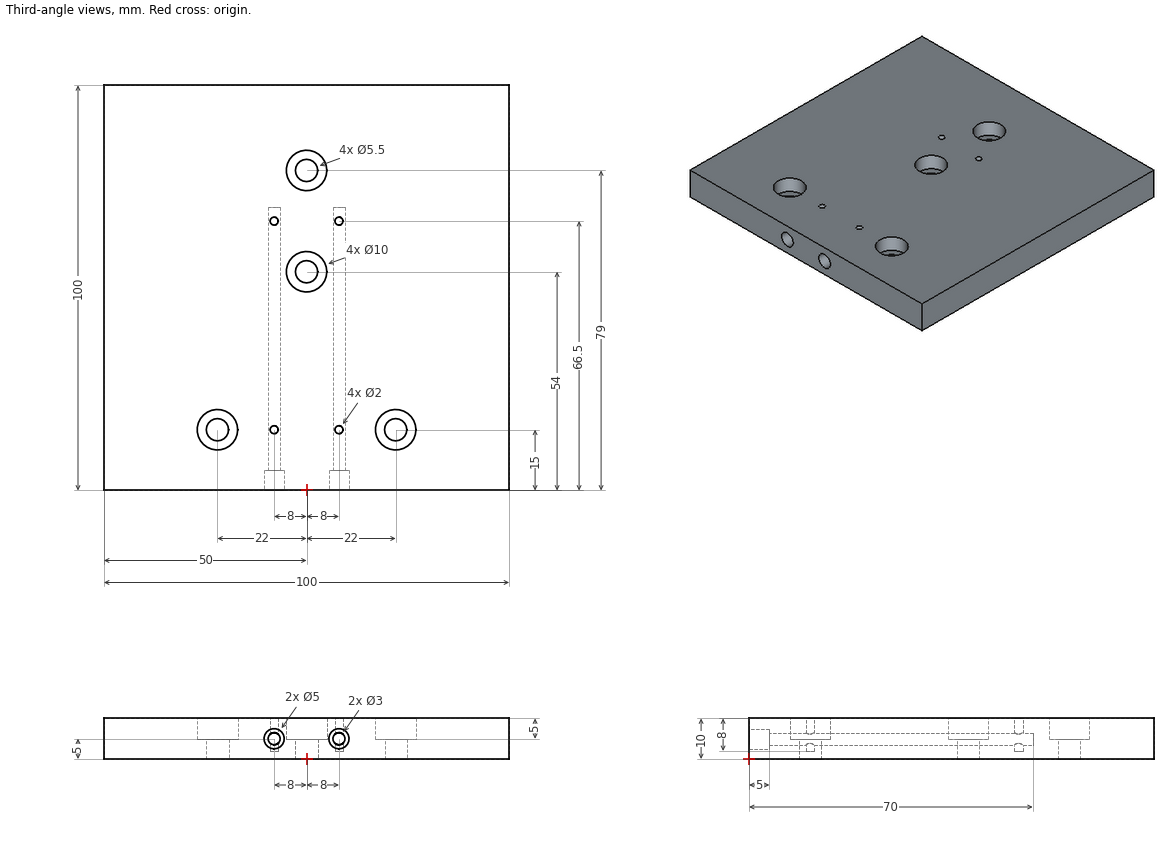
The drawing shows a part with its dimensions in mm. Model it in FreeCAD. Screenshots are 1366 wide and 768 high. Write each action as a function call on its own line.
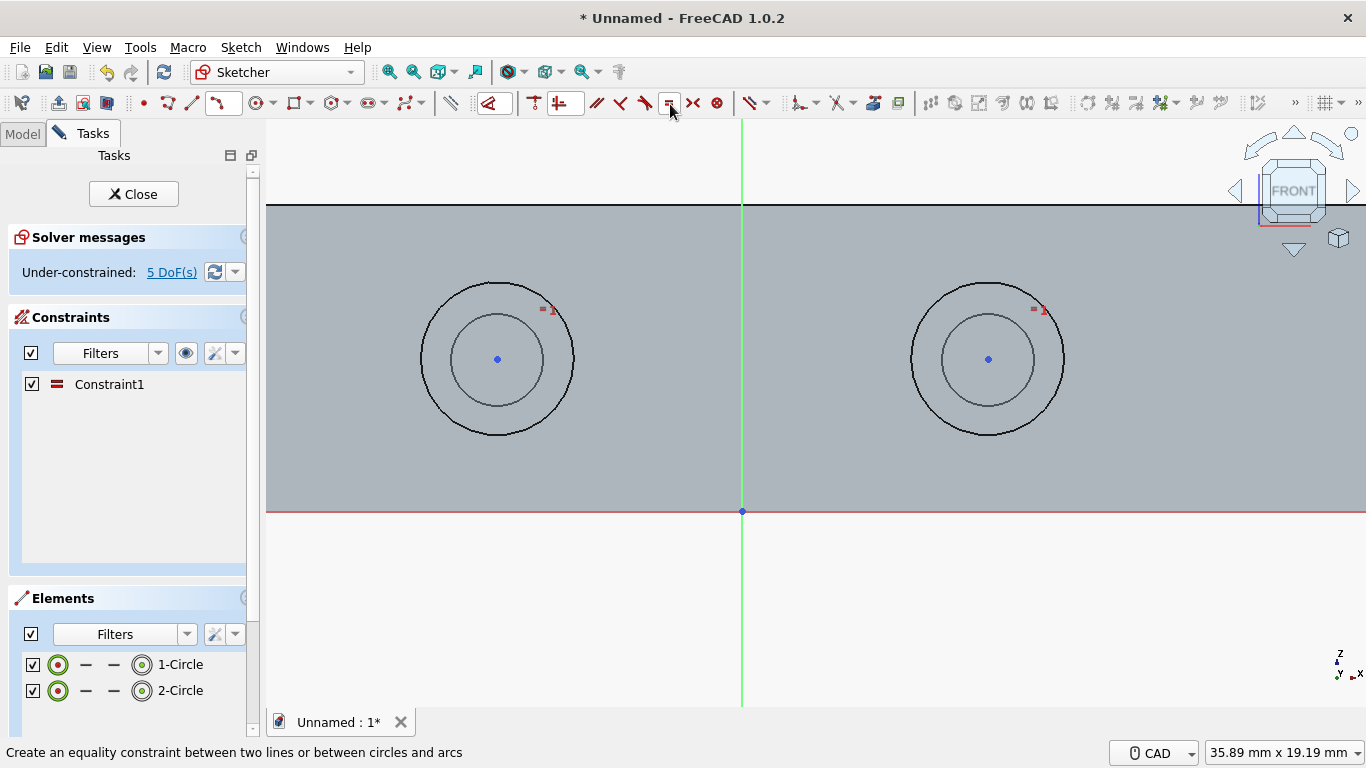
click(1020, 327)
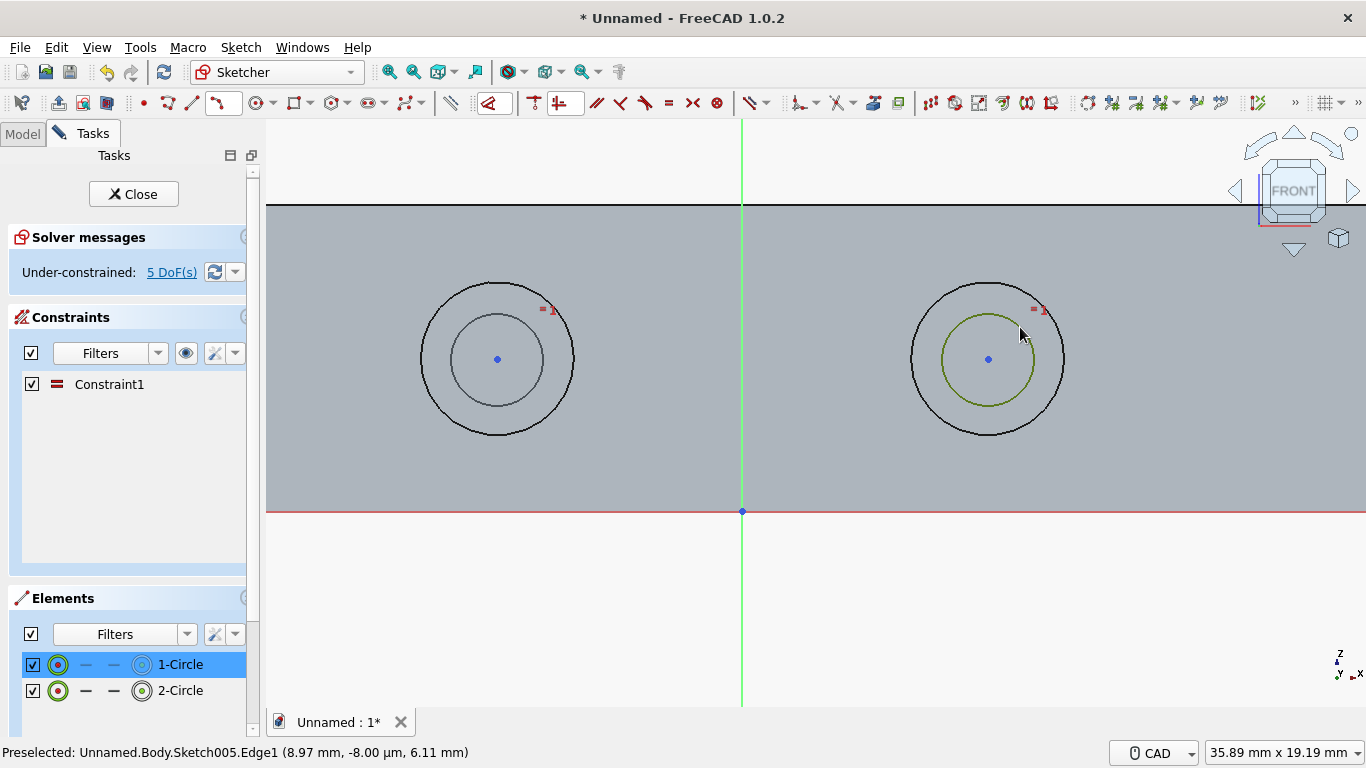
key(k)
key(o)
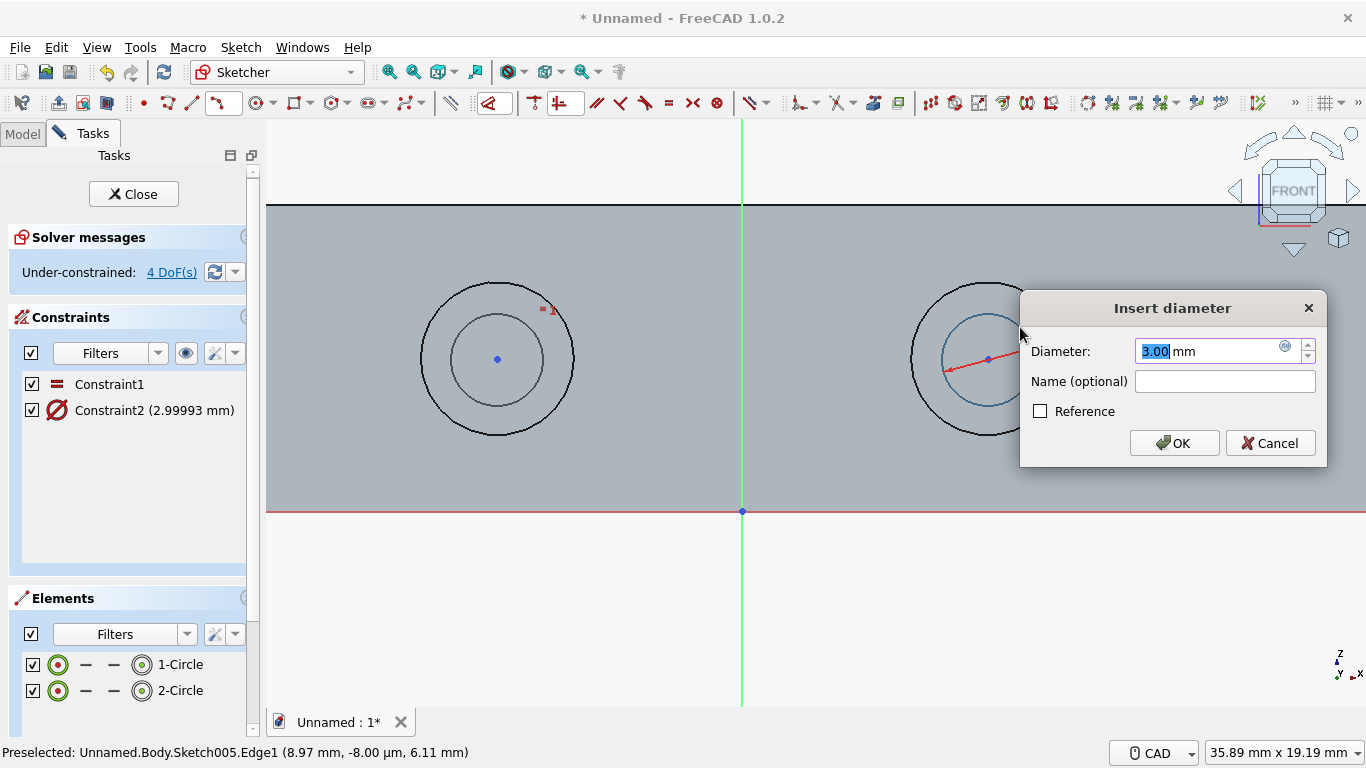
text(3)
key(Return)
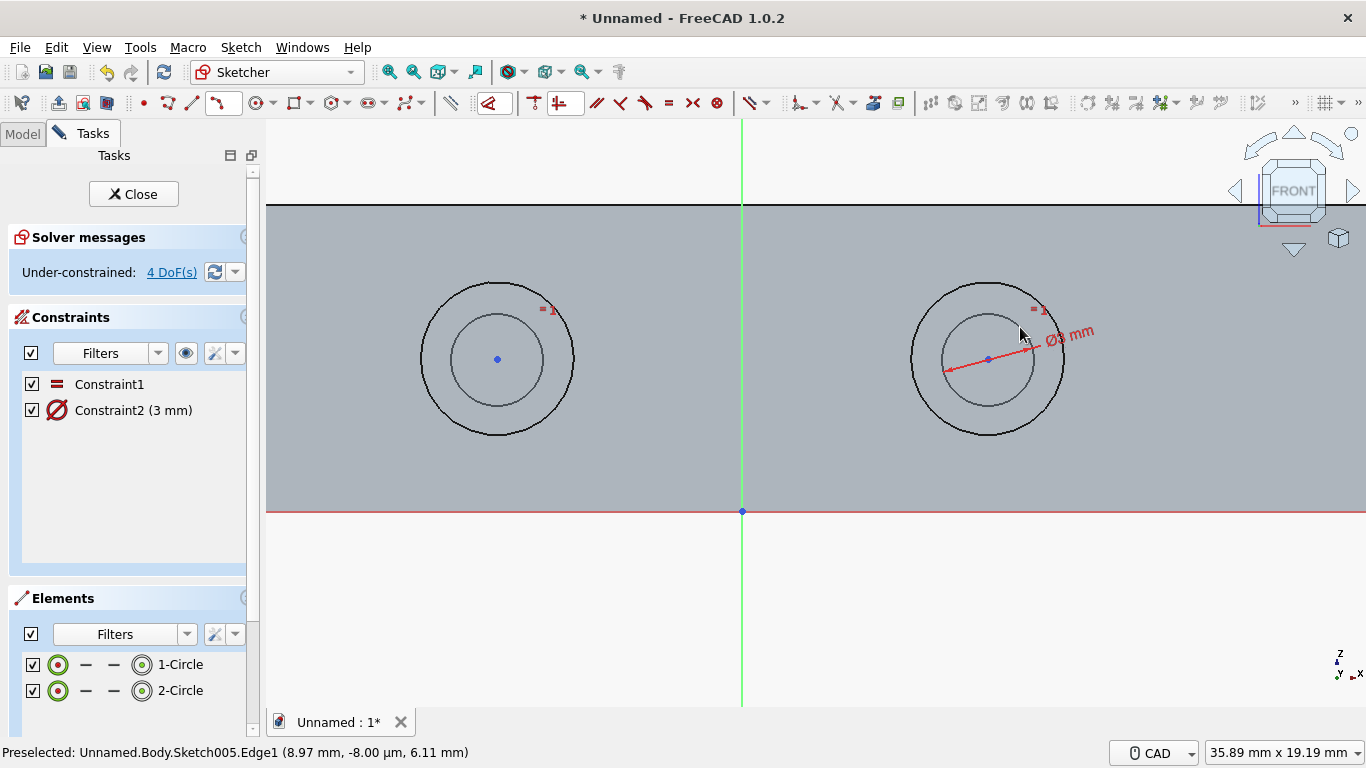
click(988, 360)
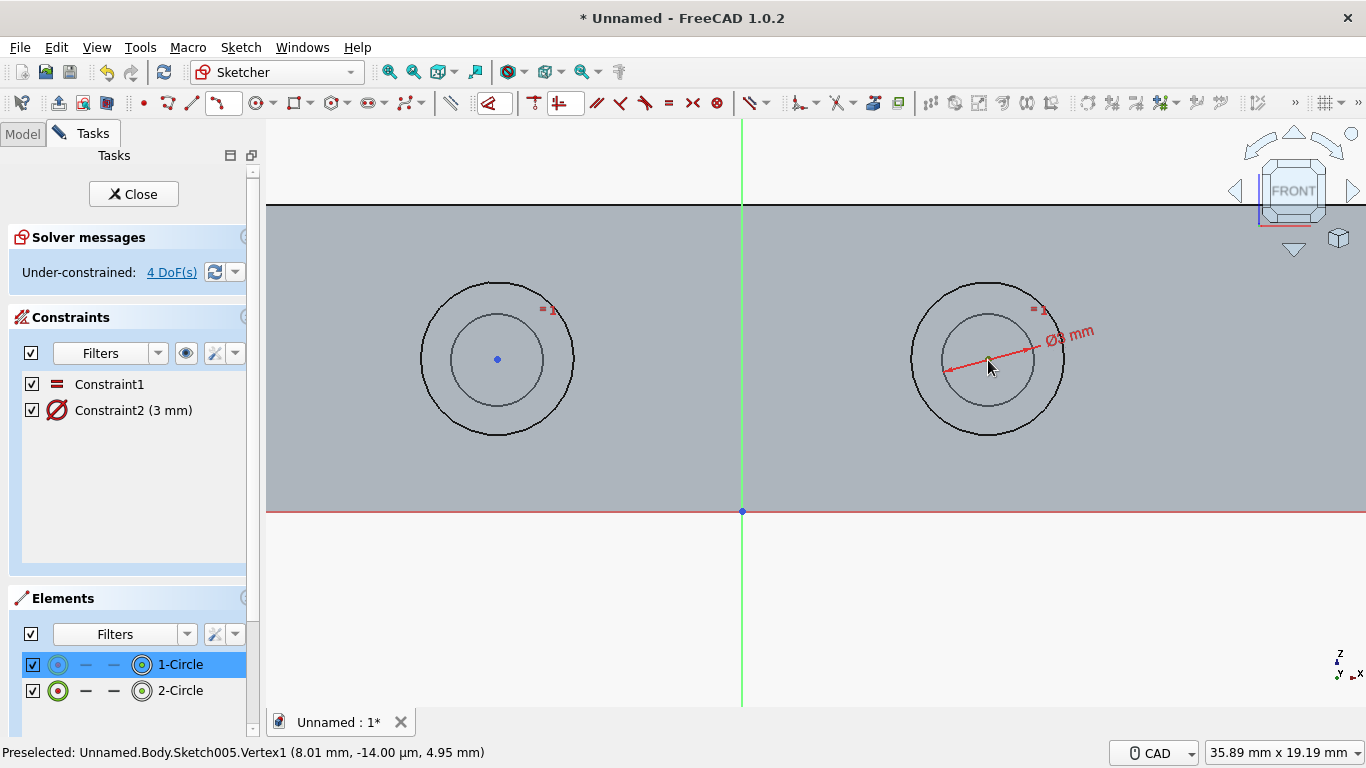
key(l)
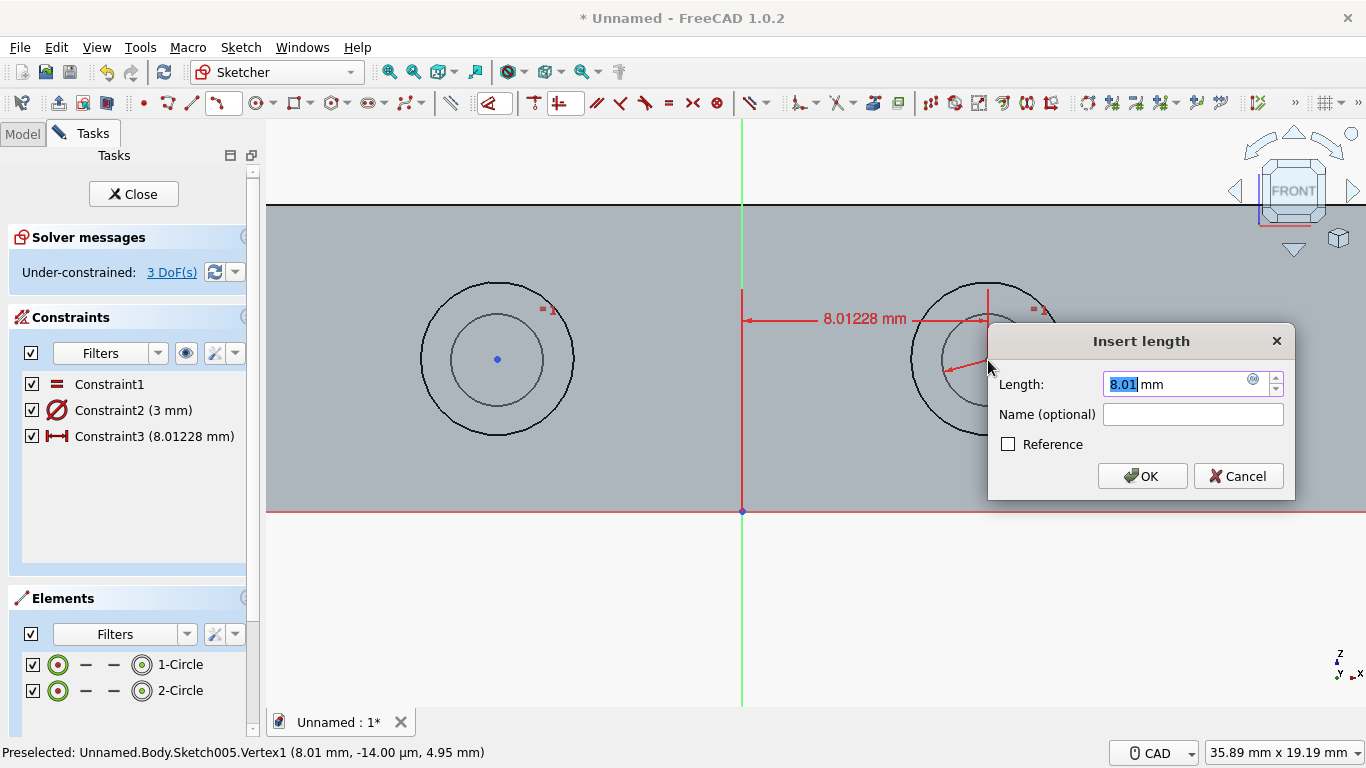
text(8)
key(Return)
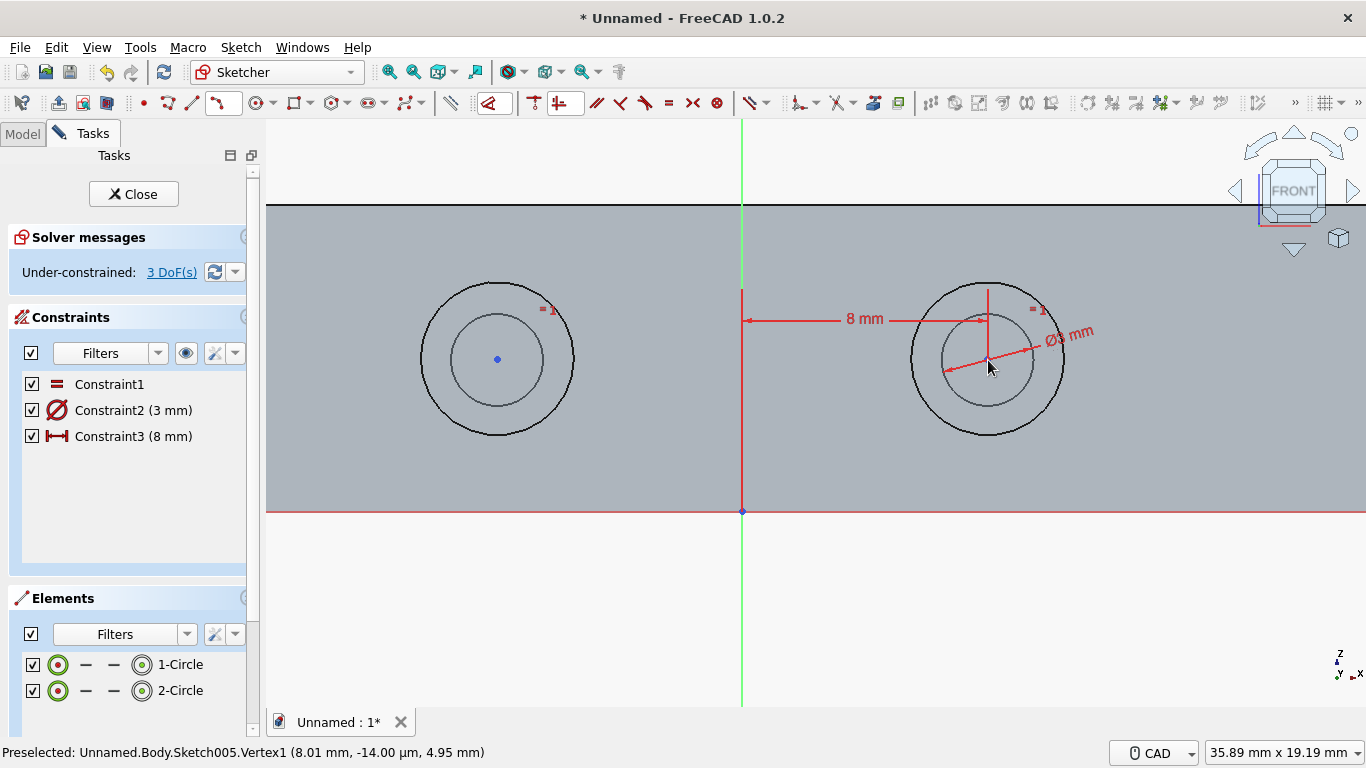
click(988, 360)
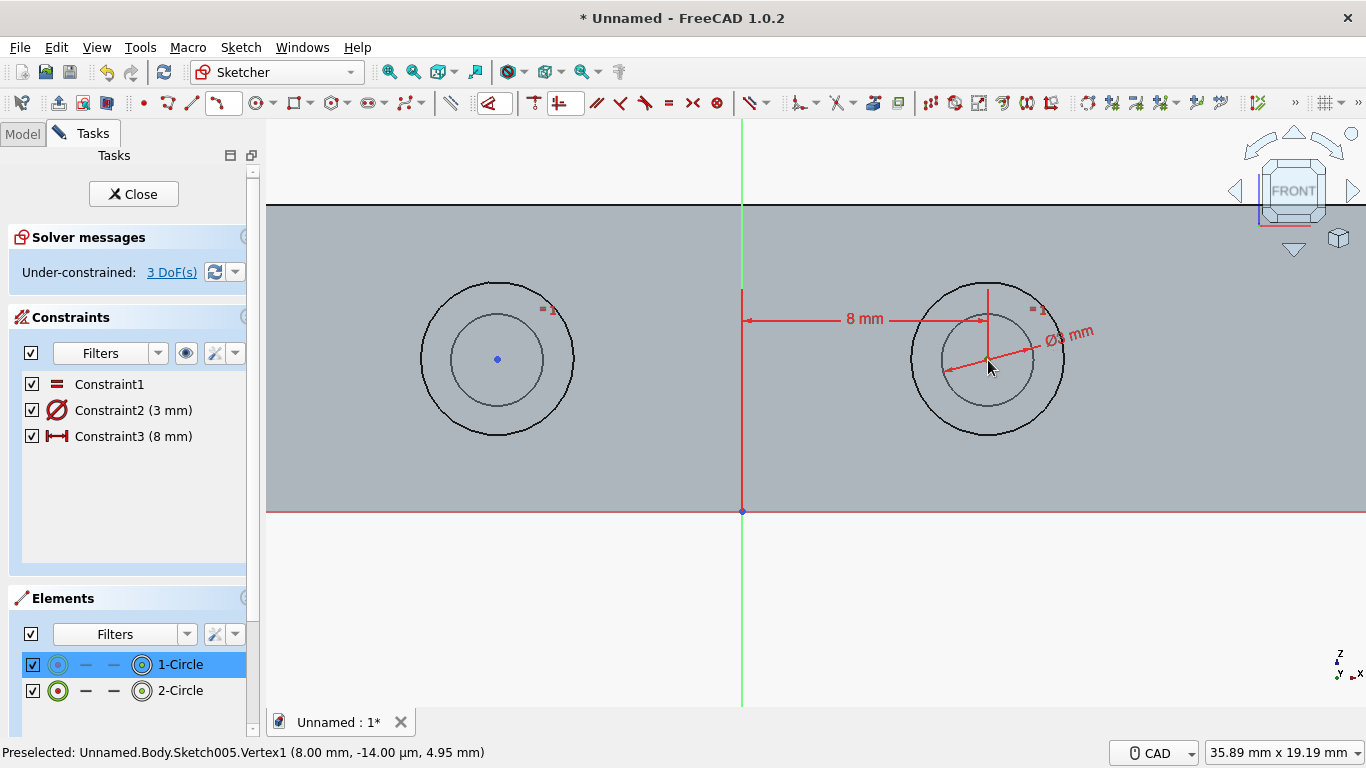
click(506, 104)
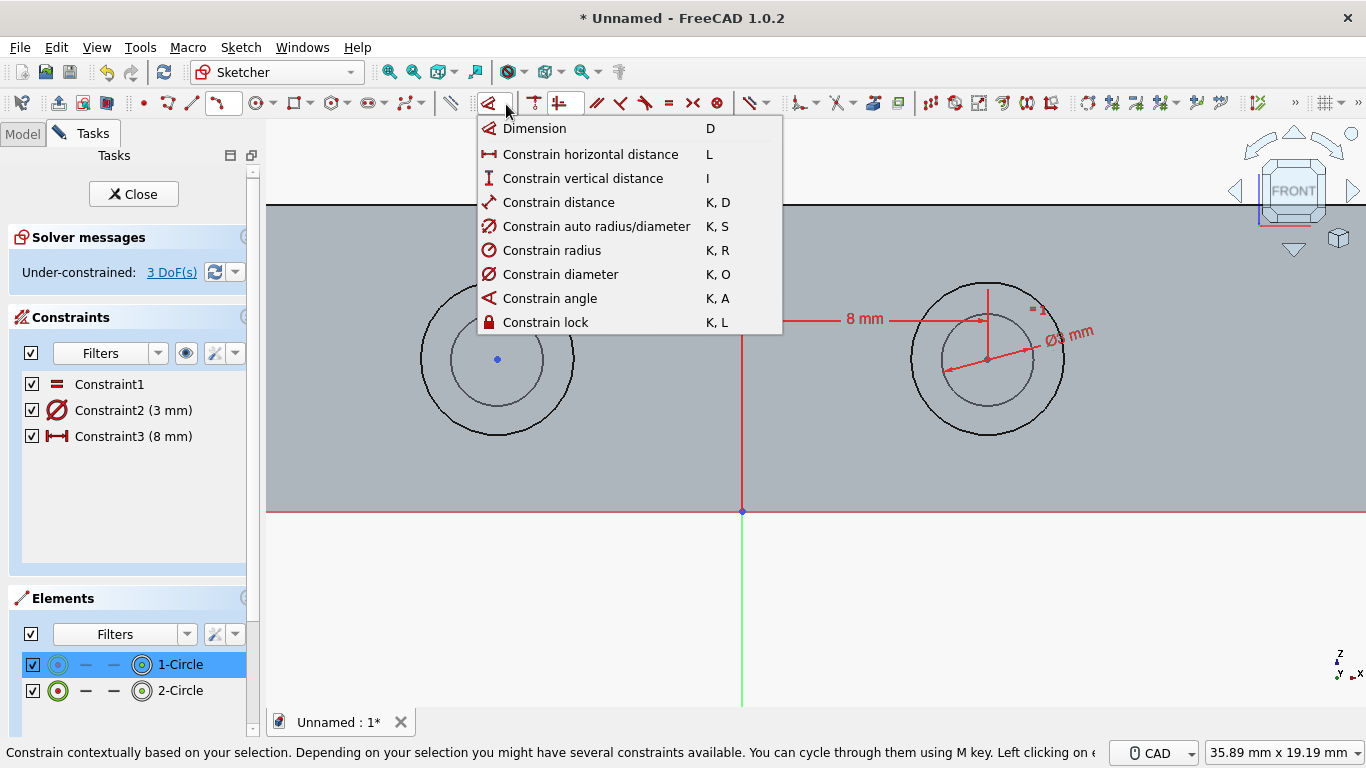
click(630, 178)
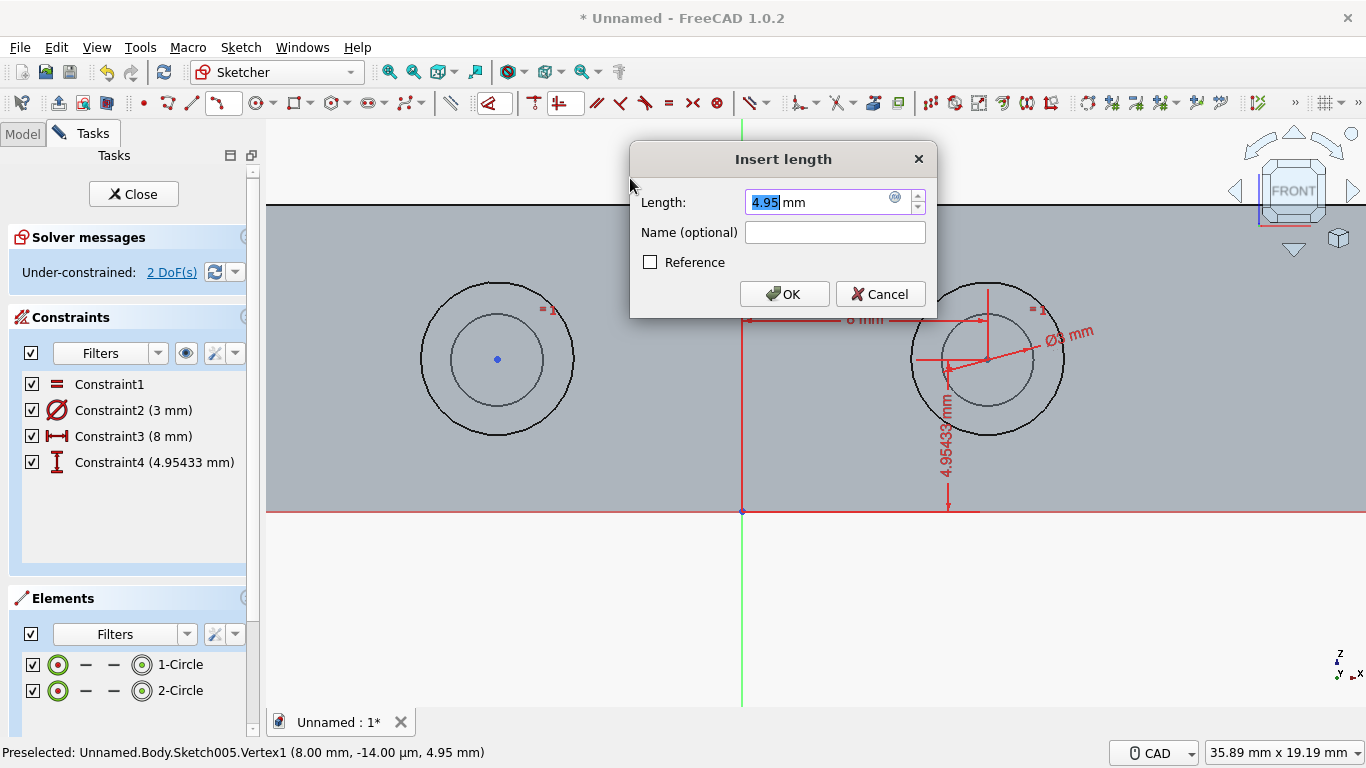
text(5)
key(Return)